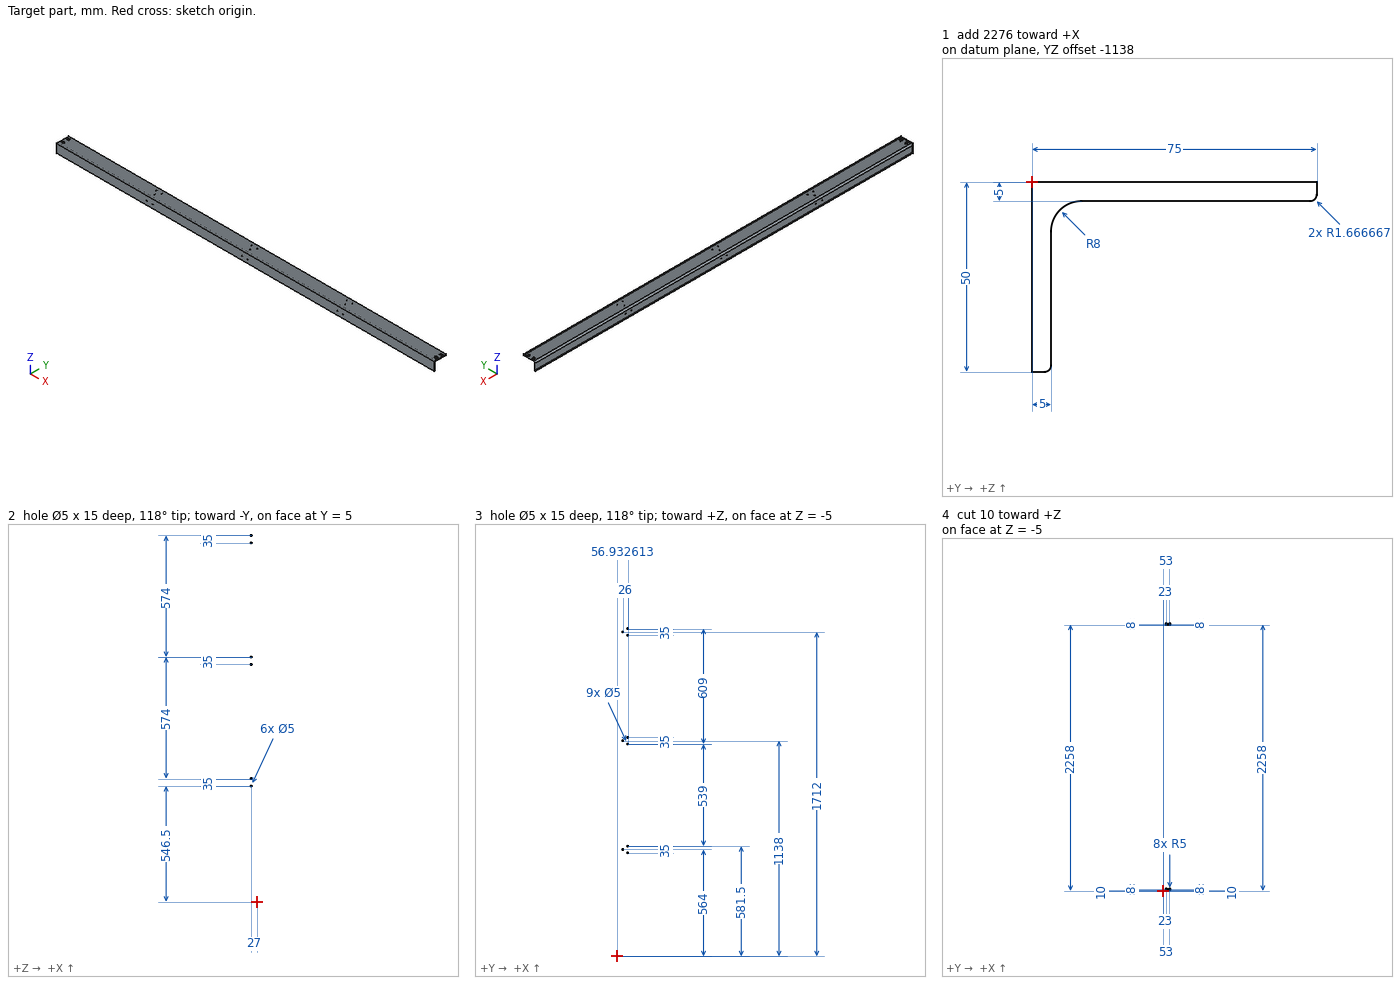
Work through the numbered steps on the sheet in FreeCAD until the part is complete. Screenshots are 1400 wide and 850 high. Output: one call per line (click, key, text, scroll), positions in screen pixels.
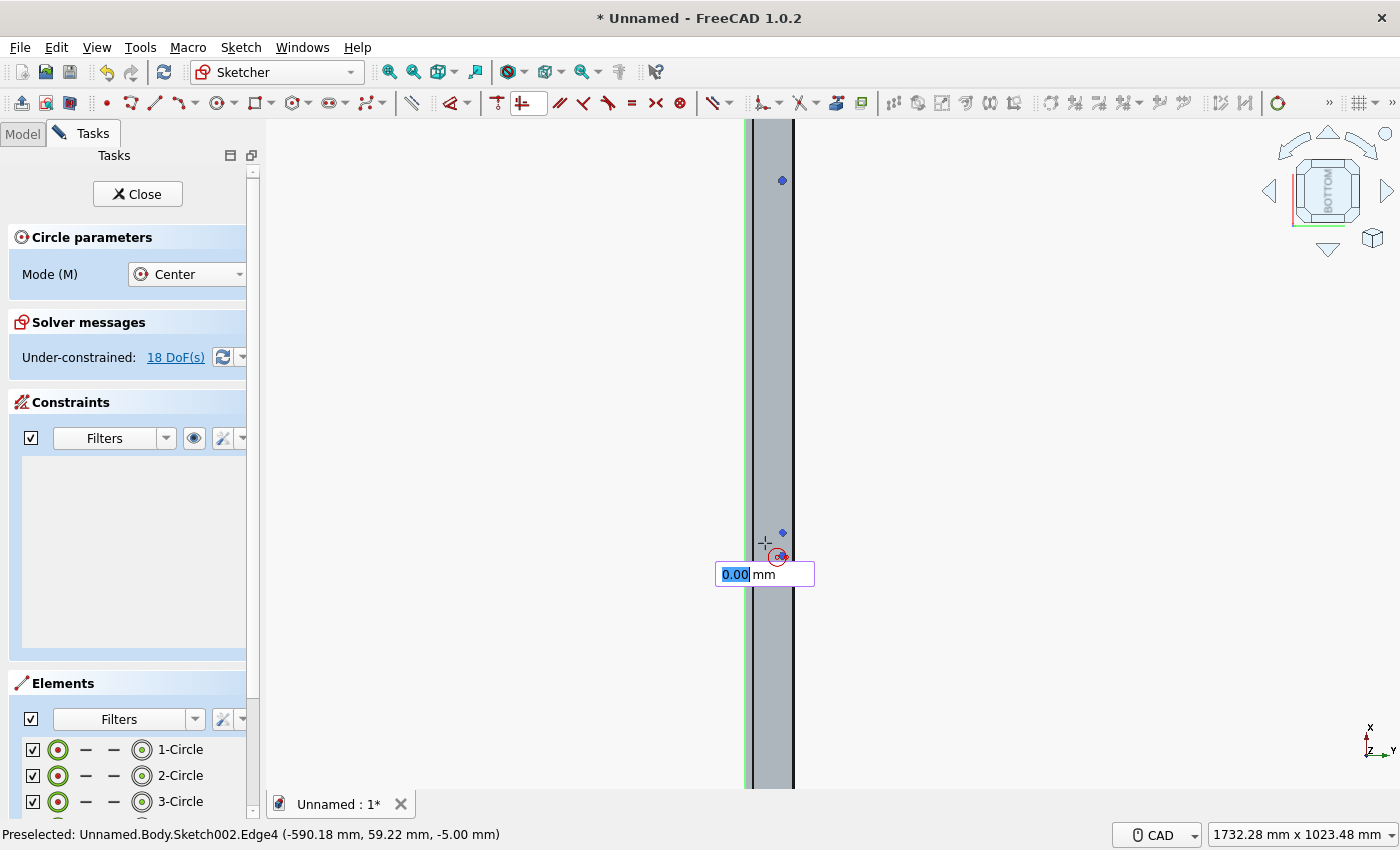
scroll(766, 541, up, 12)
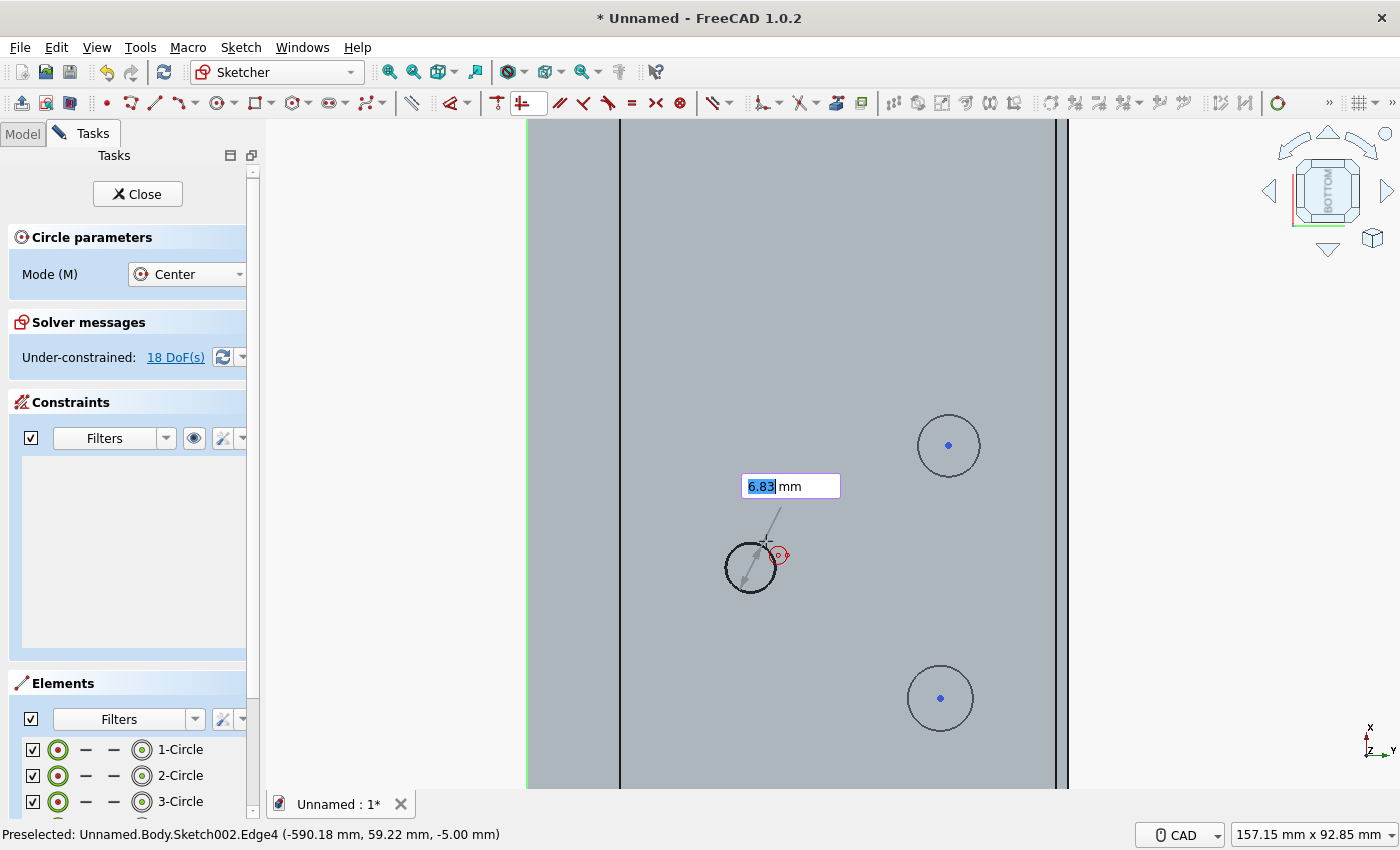
click(763, 540)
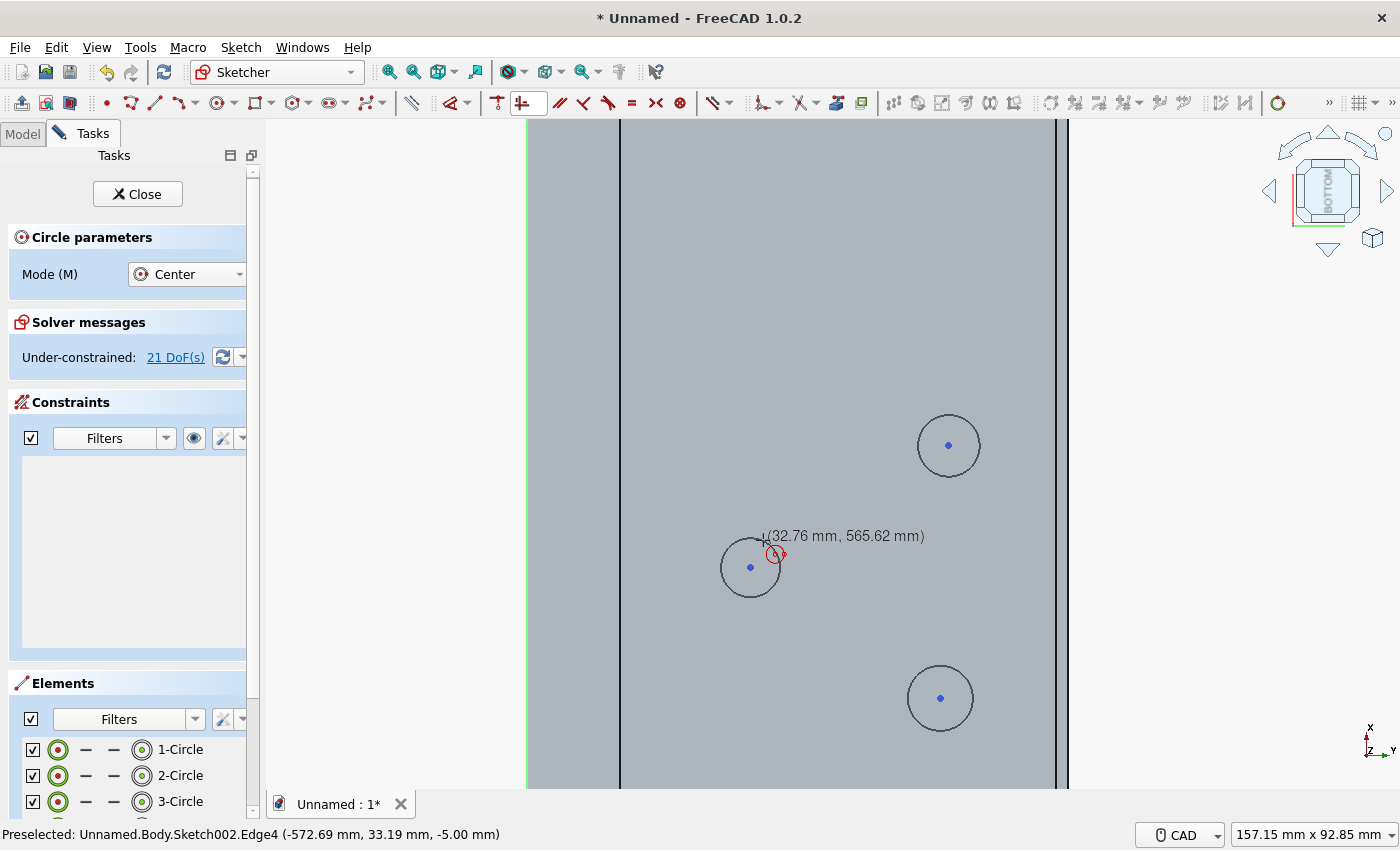
scroll(765, 542, down, 16)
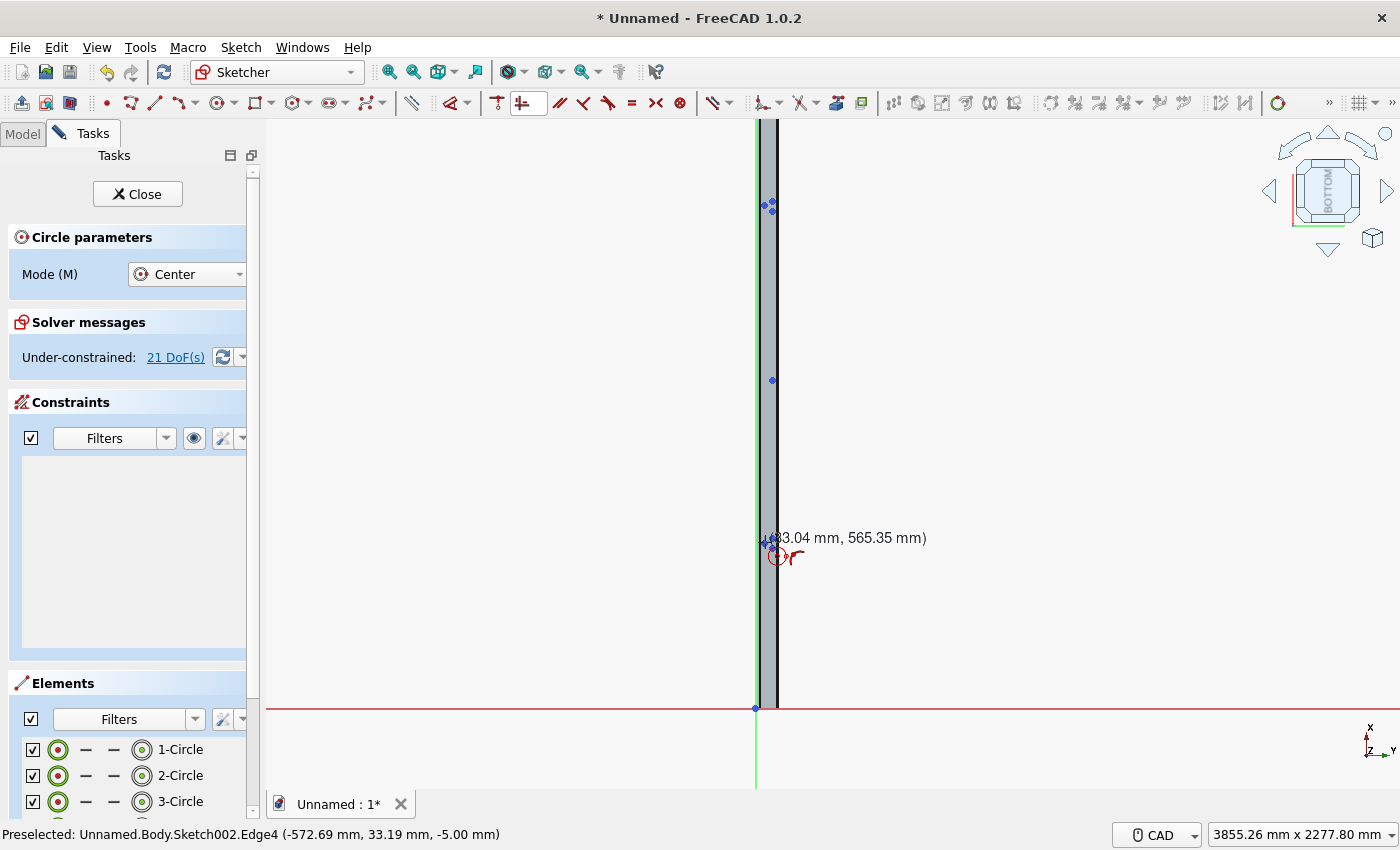
scroll(772, 369, up, 18)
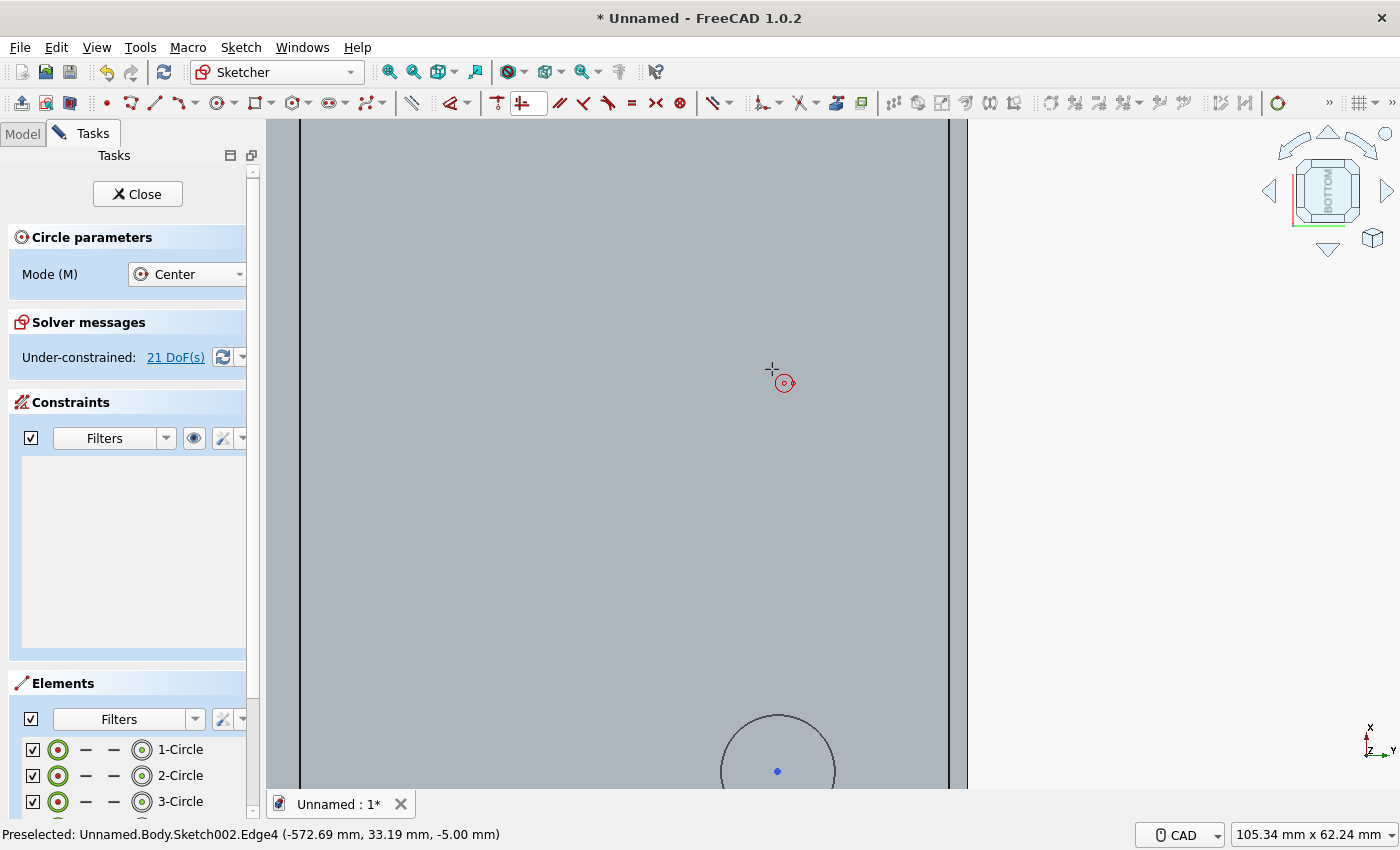
scroll(773, 369, down, 18)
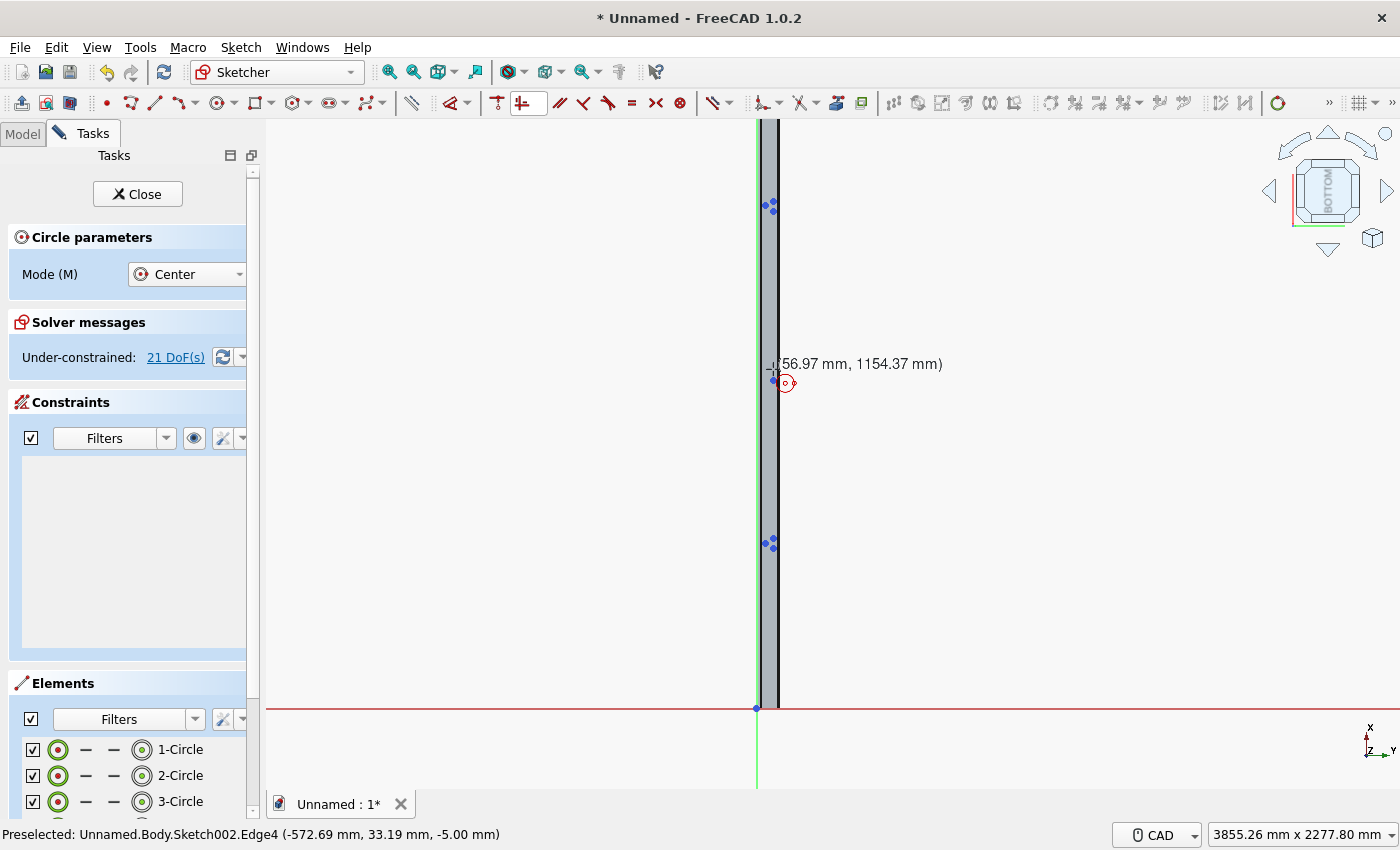
scroll(773, 369, up, 3)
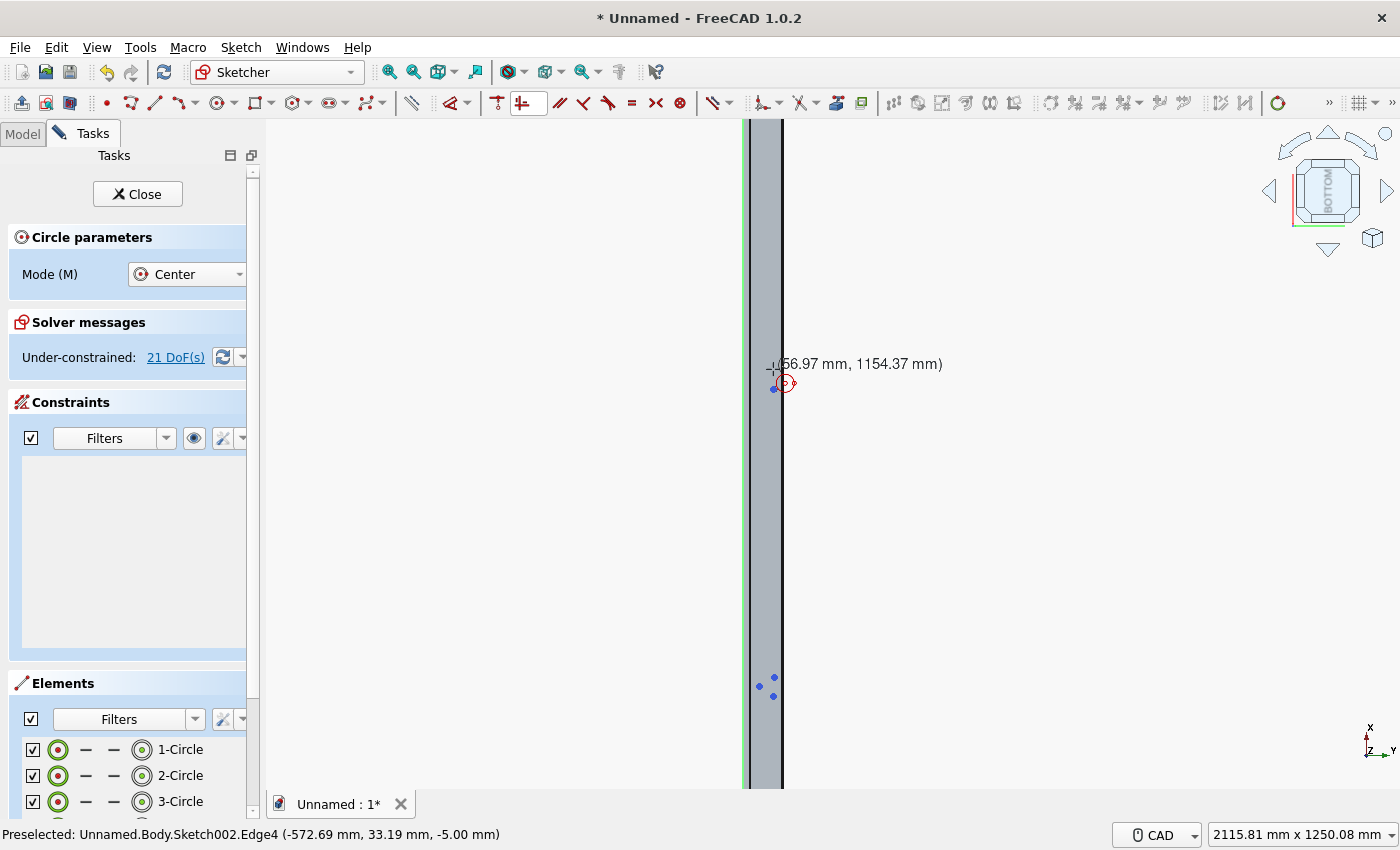
click(773, 369)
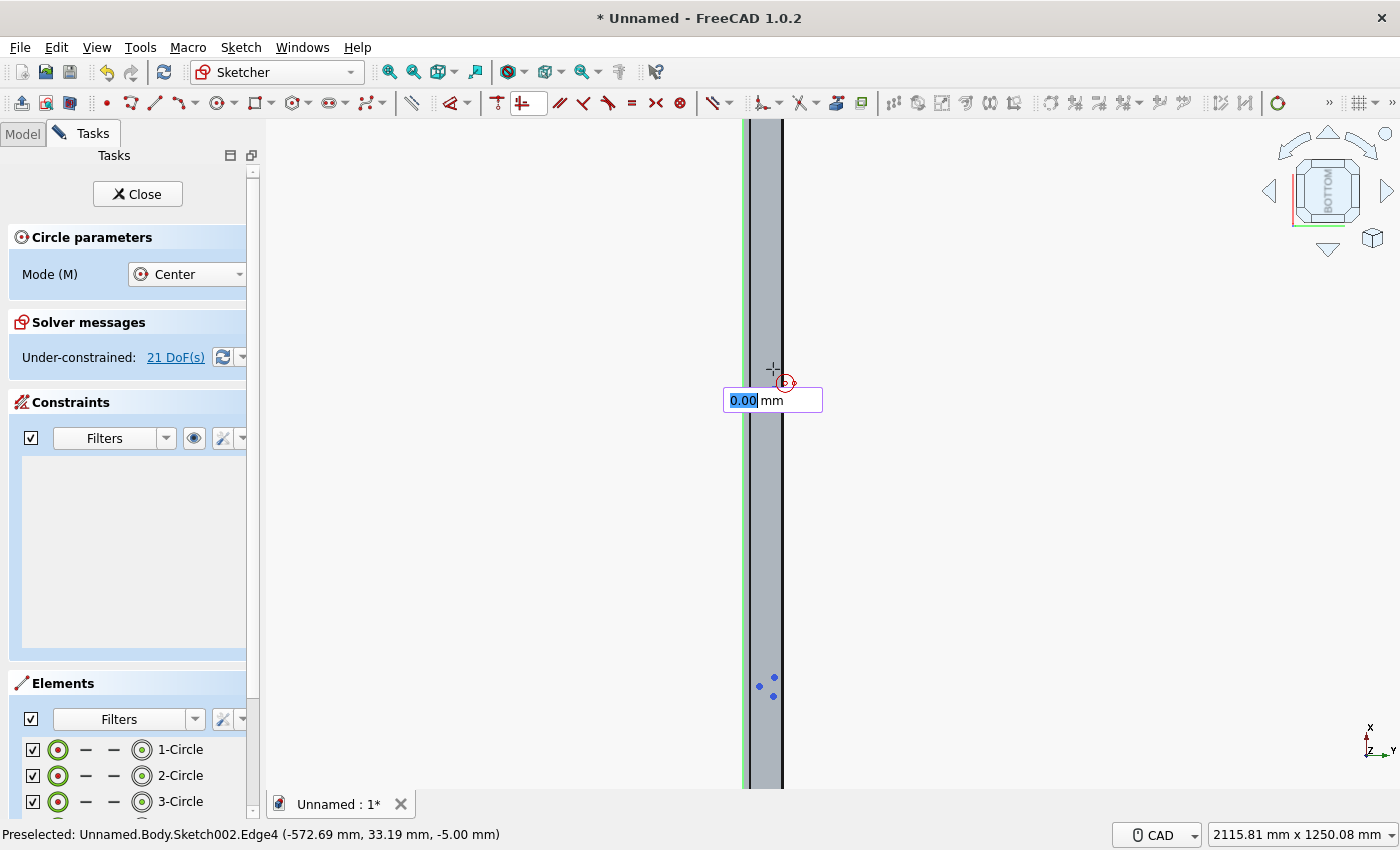
scroll(774, 368, up, 13)